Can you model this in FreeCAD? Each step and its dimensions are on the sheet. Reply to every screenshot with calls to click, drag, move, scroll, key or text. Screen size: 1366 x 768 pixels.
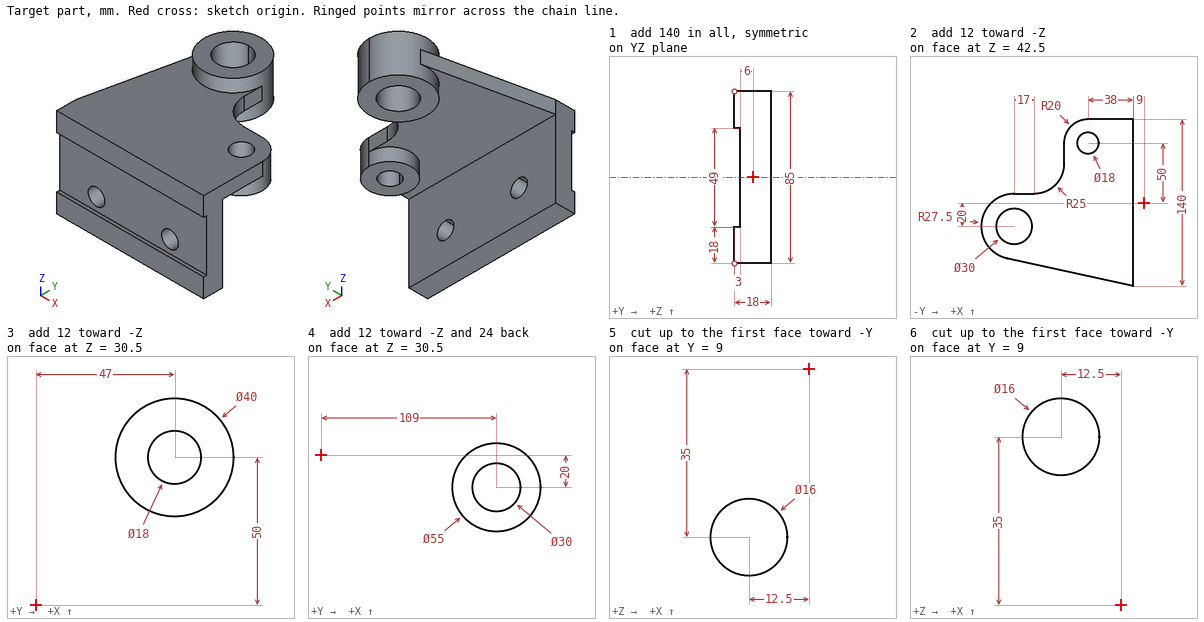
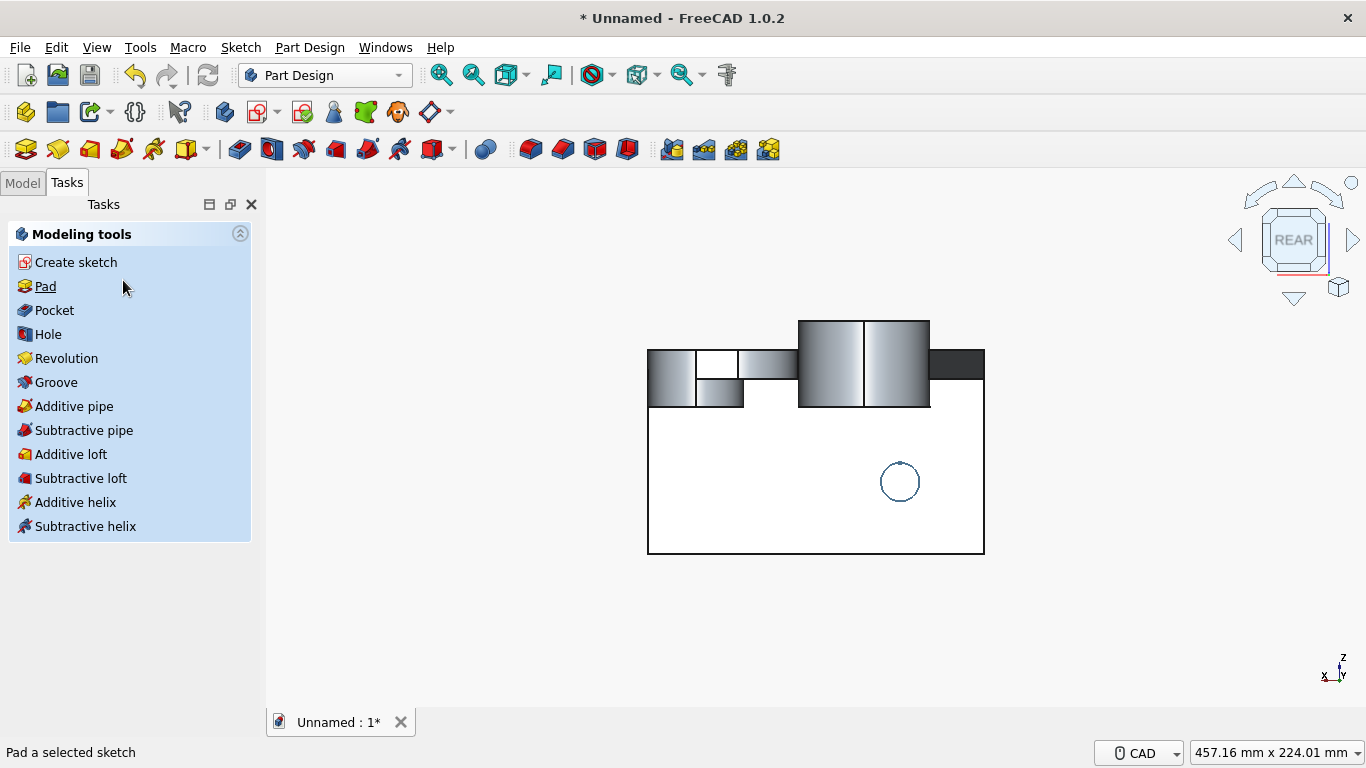
click(240, 150)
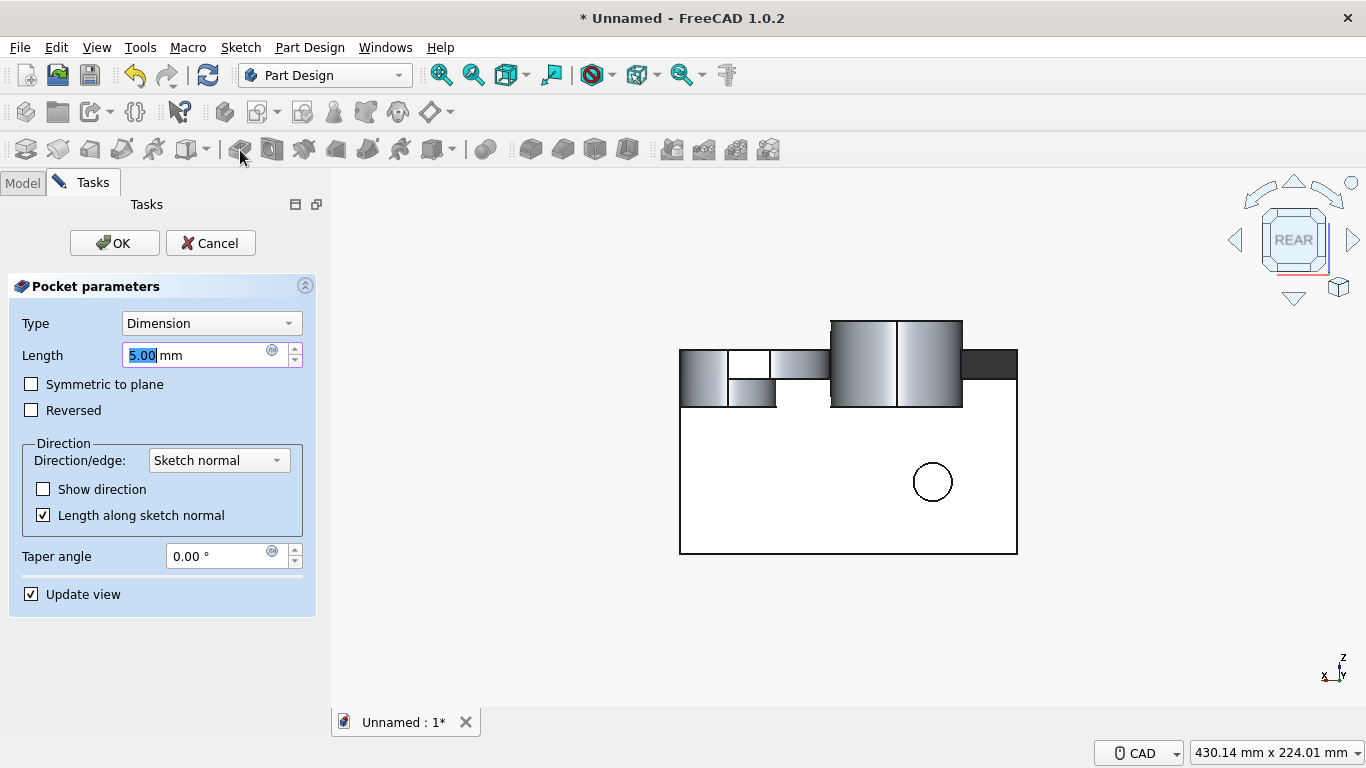
click(212, 324)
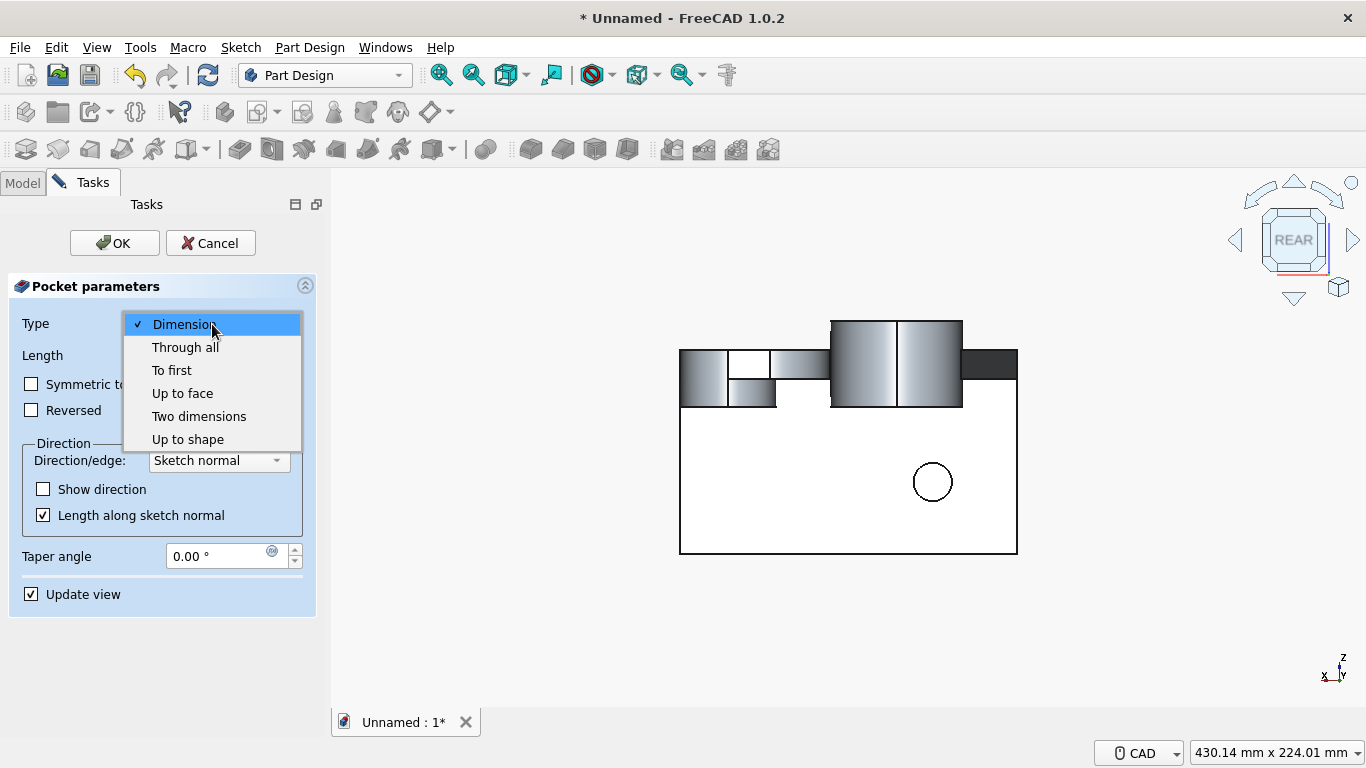
click(212, 370)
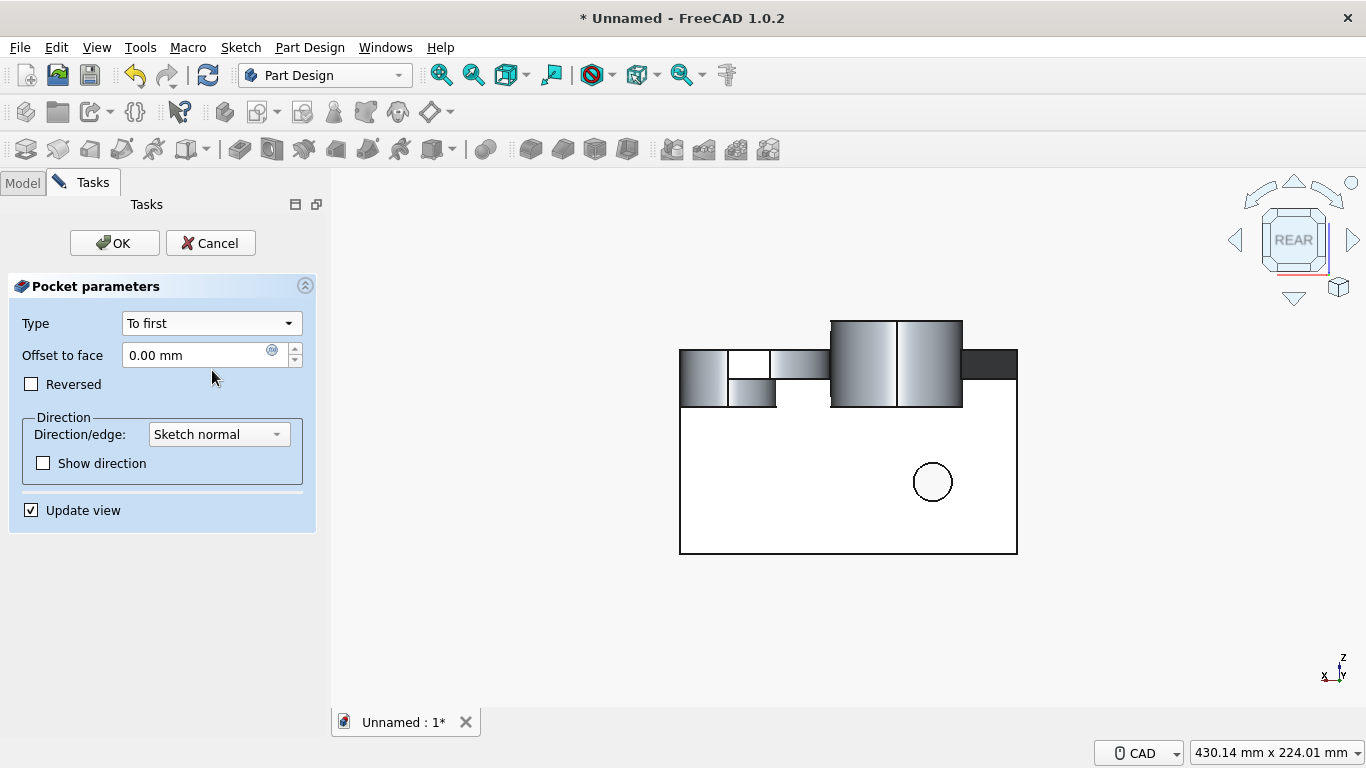
click(115, 243)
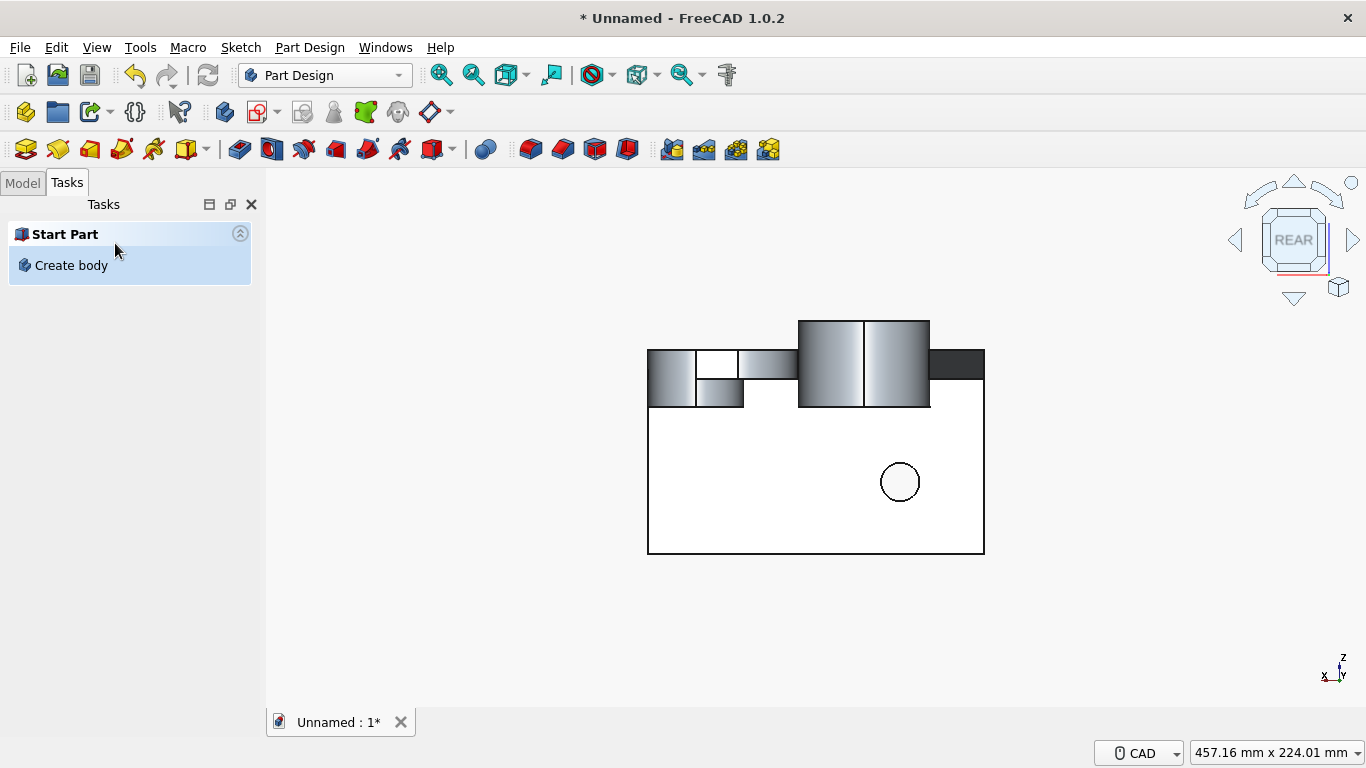
click(442, 76)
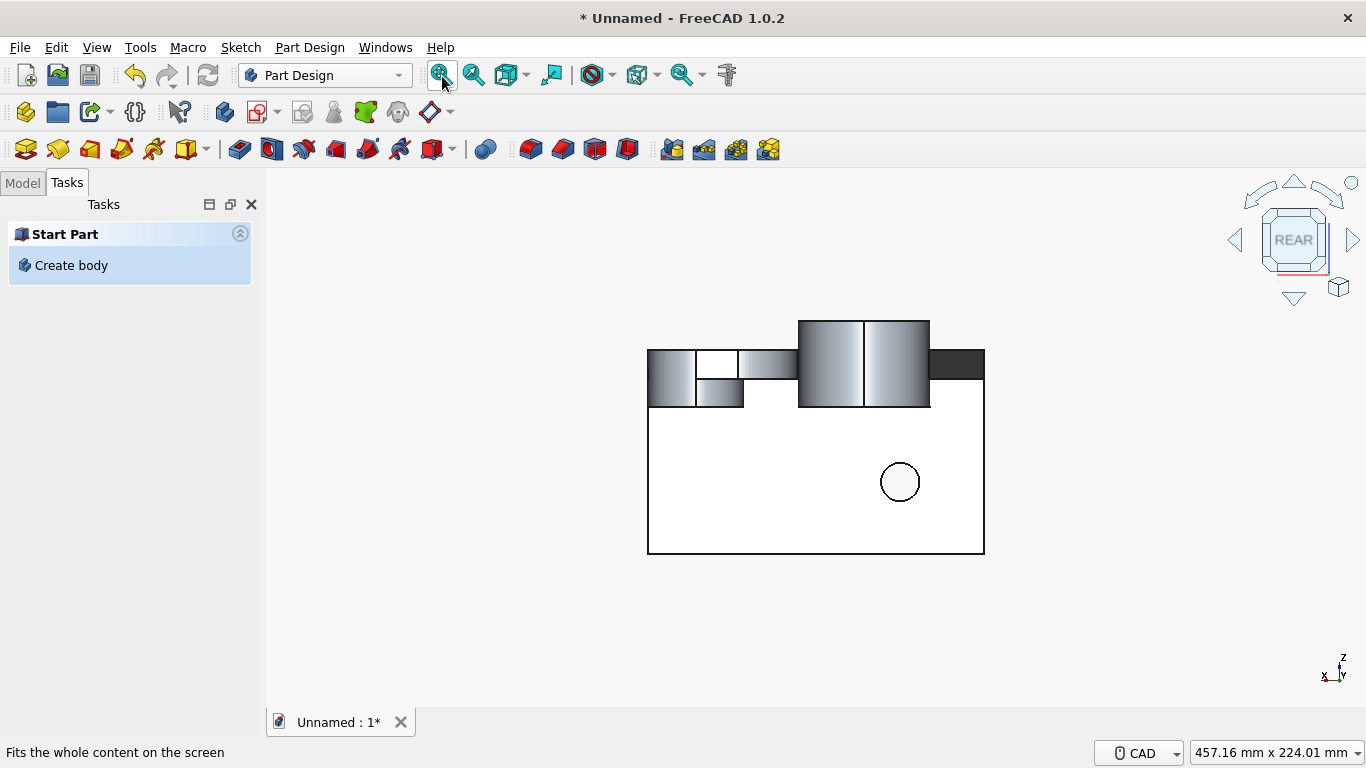
click(768, 465)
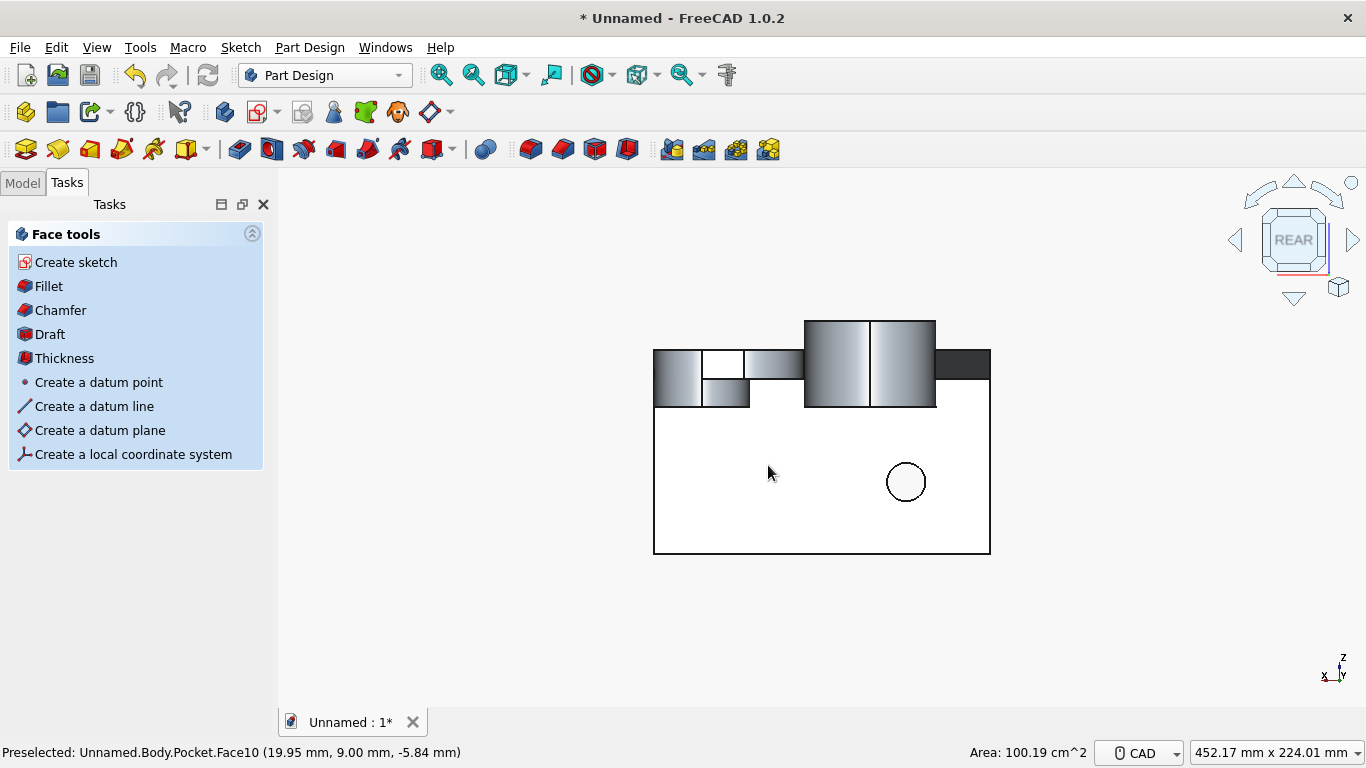
click(258, 112)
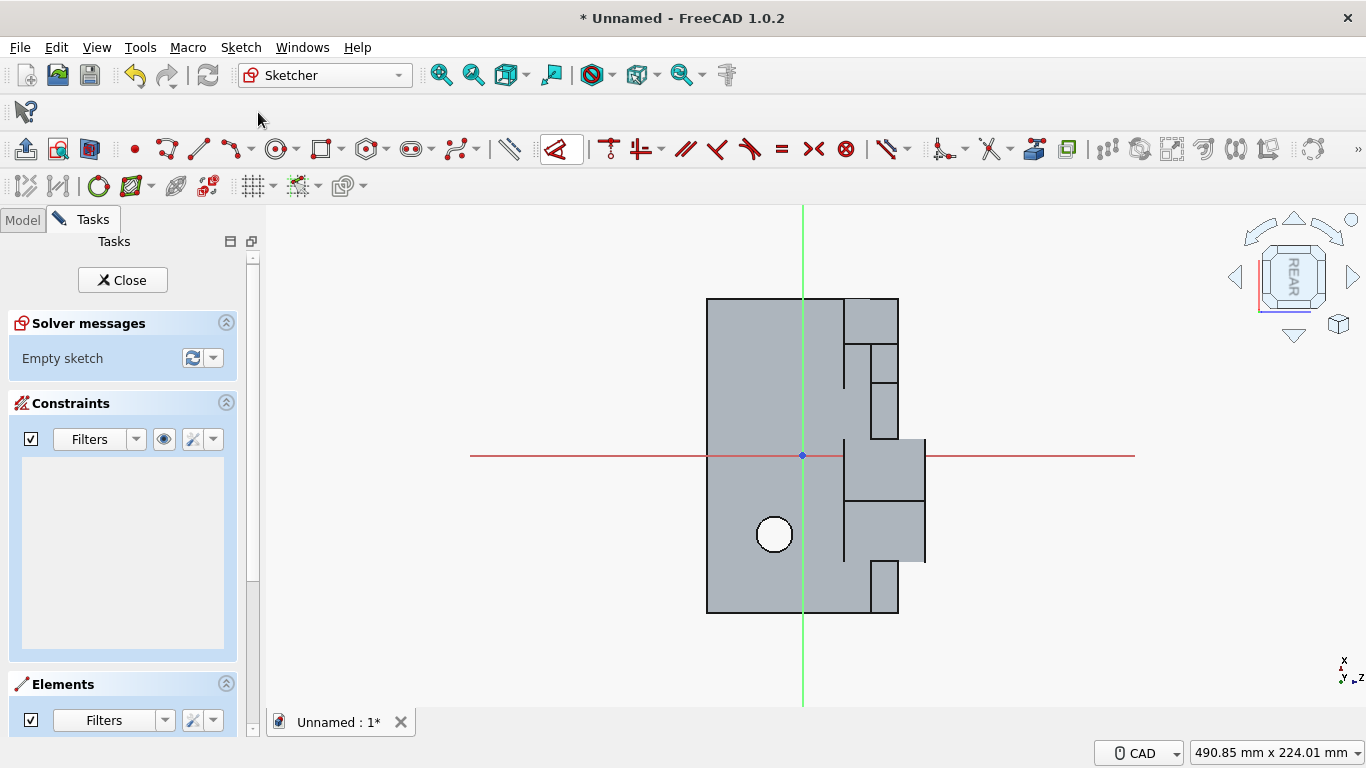
scroll(778, 368, up, 11)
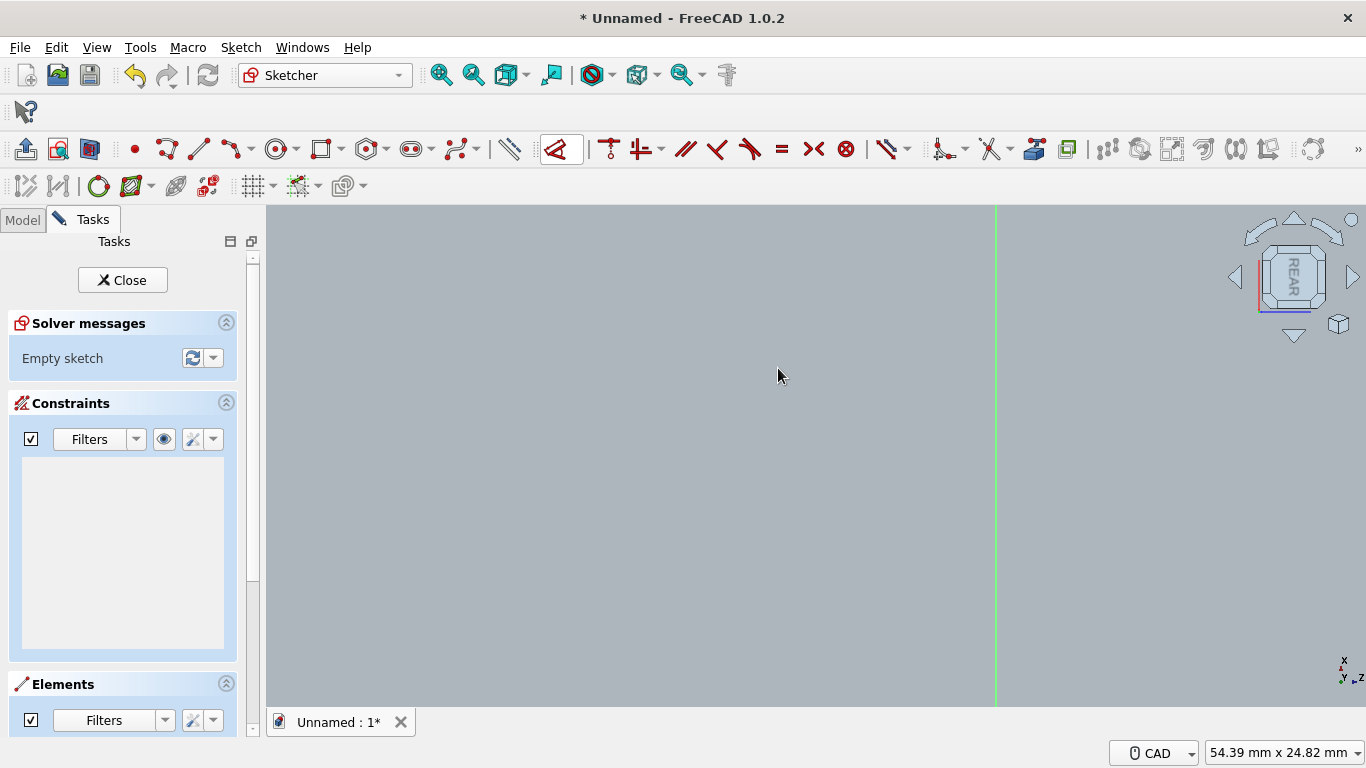
key(g)
key(c)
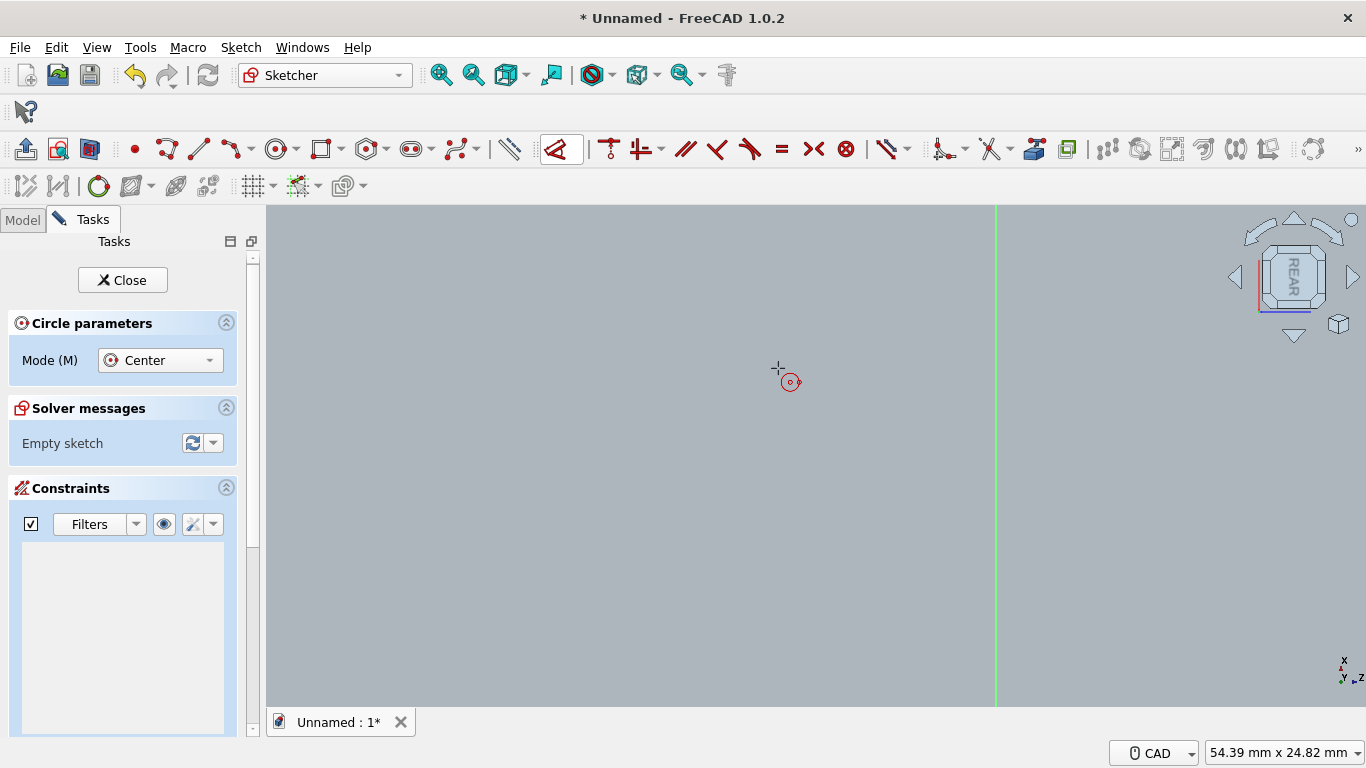
click(743, 452)
move(857, 337)